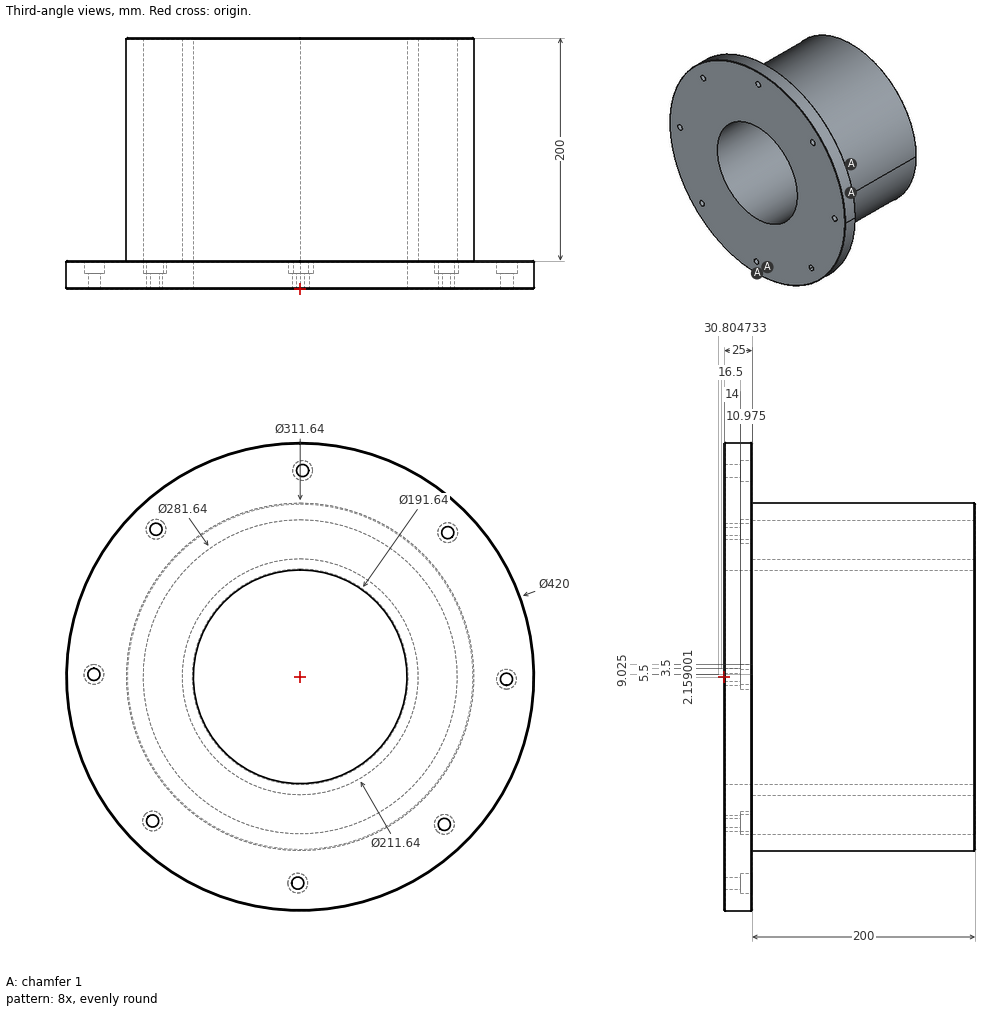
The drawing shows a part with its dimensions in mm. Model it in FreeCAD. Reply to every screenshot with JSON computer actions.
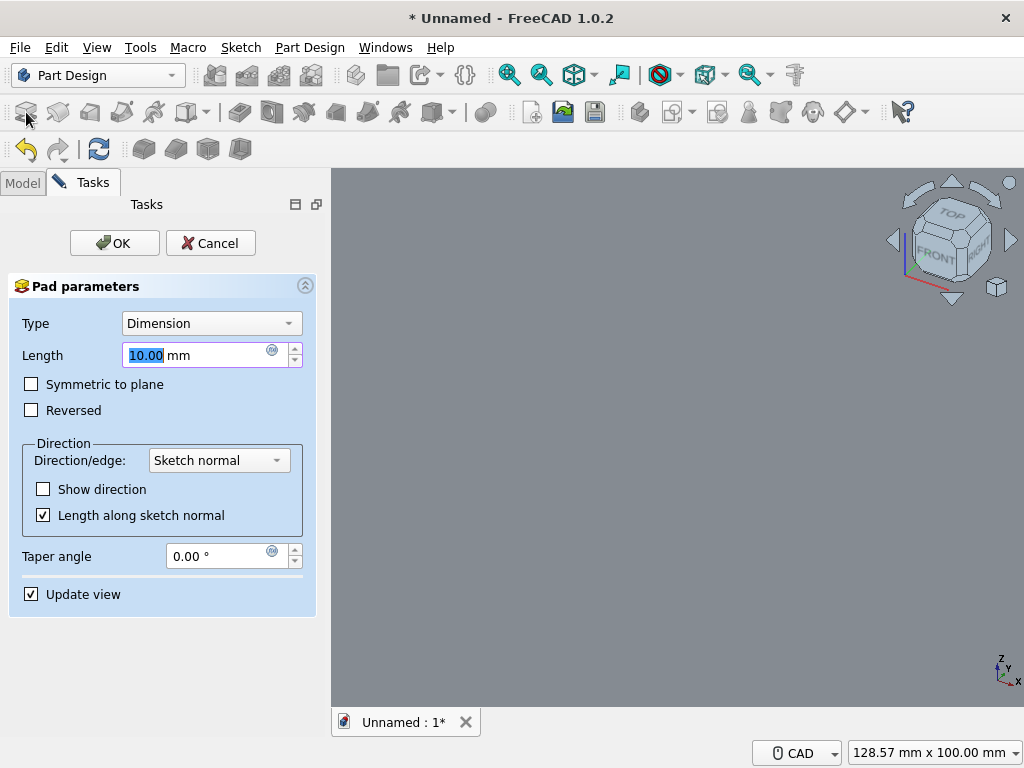
{"action": "type", "text": "25"}
{"action": "key", "text": "Tab"}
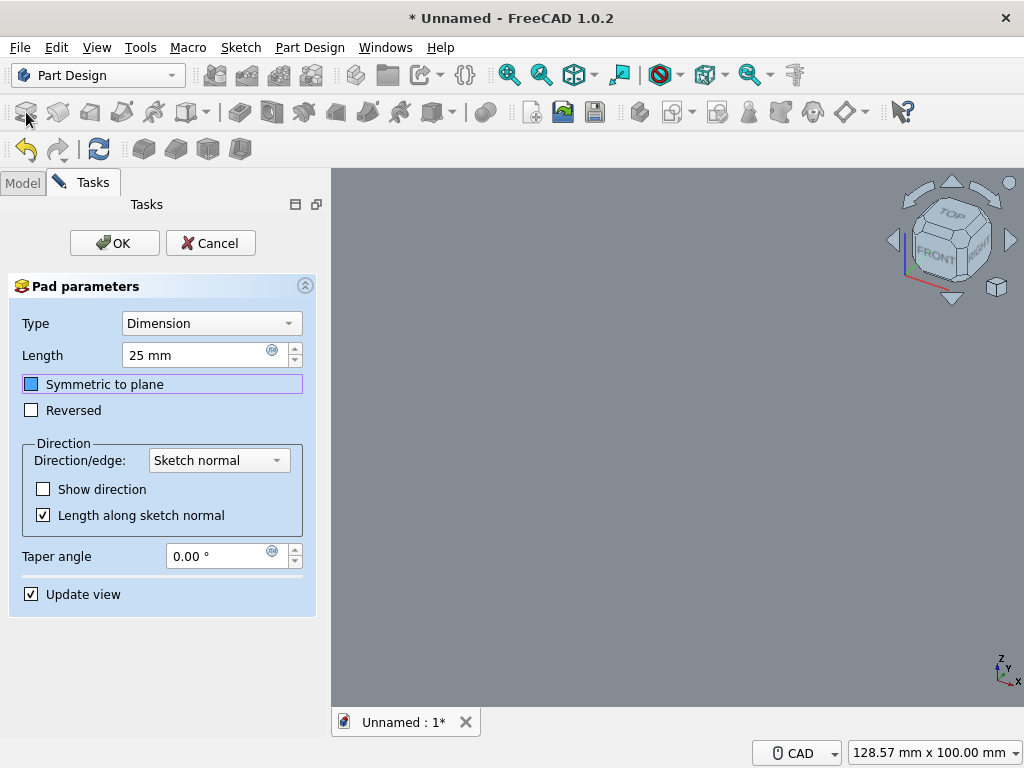
{"action": "left_click", "coordinate": [30, 410]}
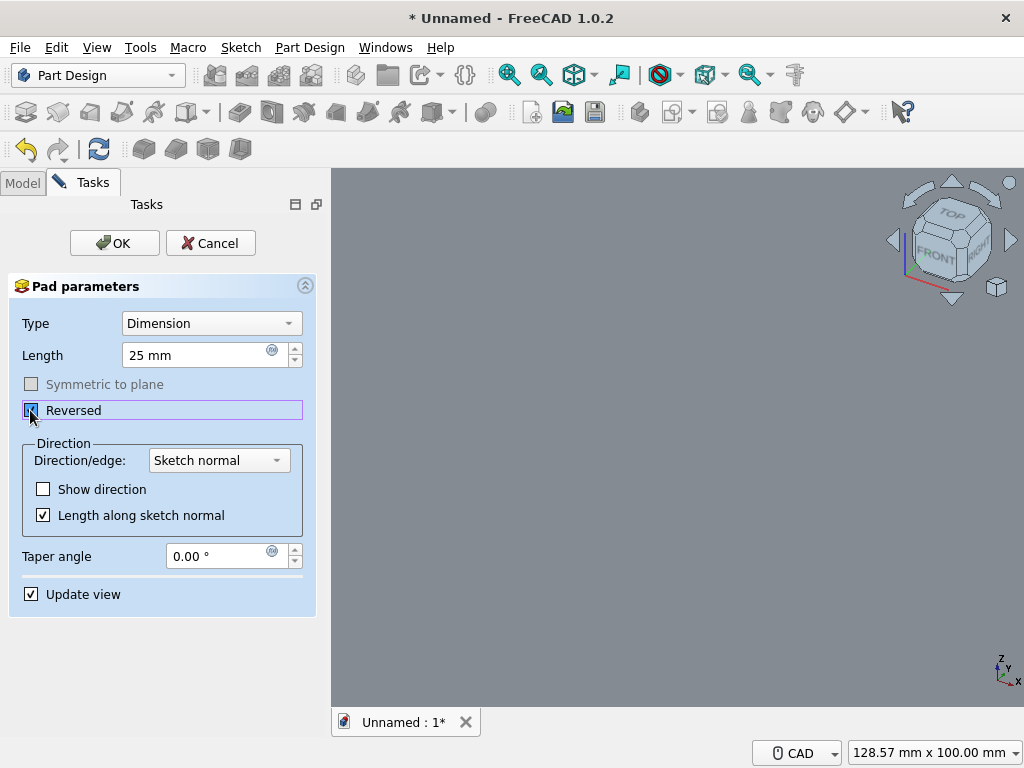
{"action": "left_click", "coordinate": [115, 243]}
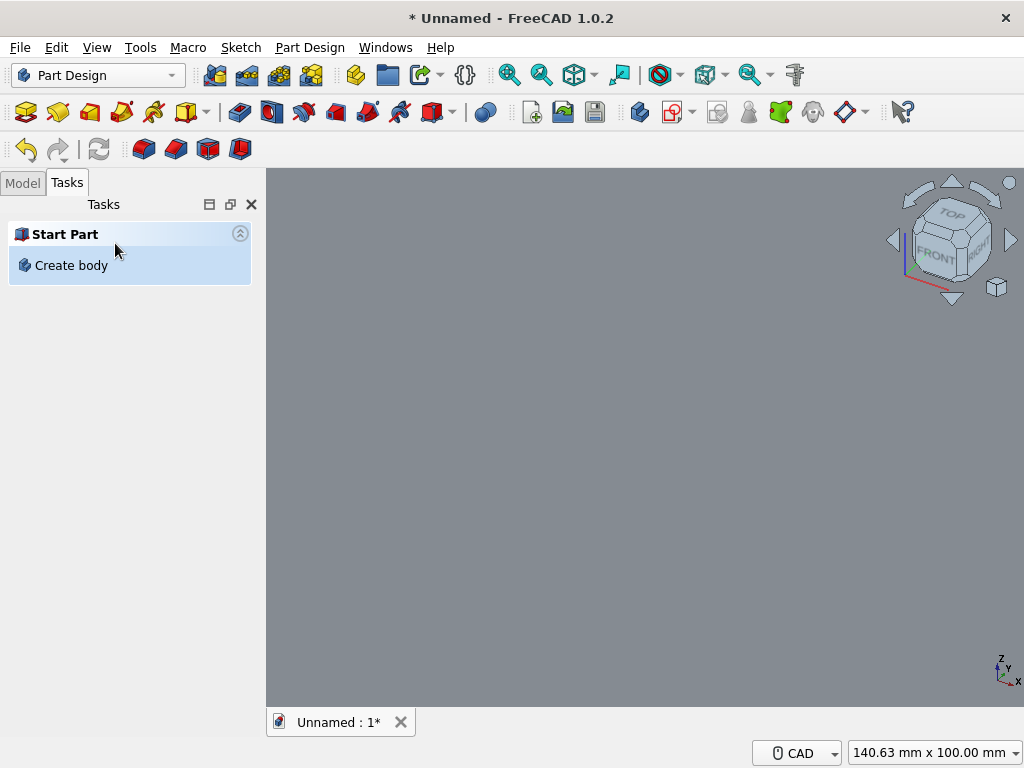
{"action": "key", "text": "v f"}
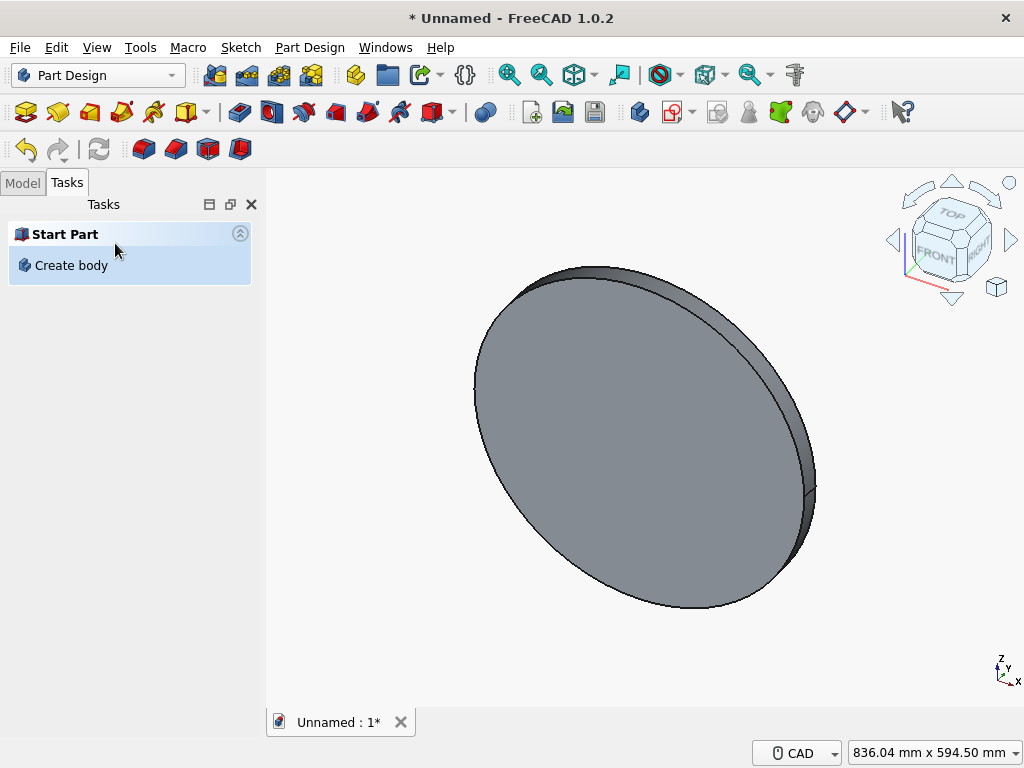
{"action": "key", "text": "4"}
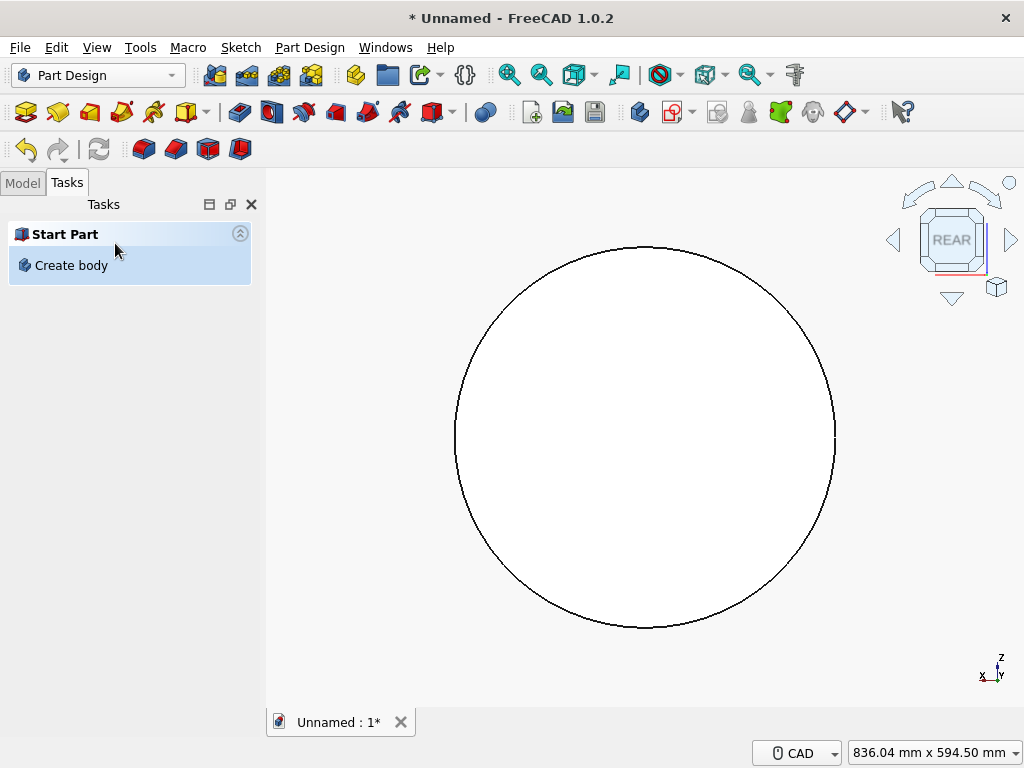
{"action": "left_click", "coordinate": [645, 436]}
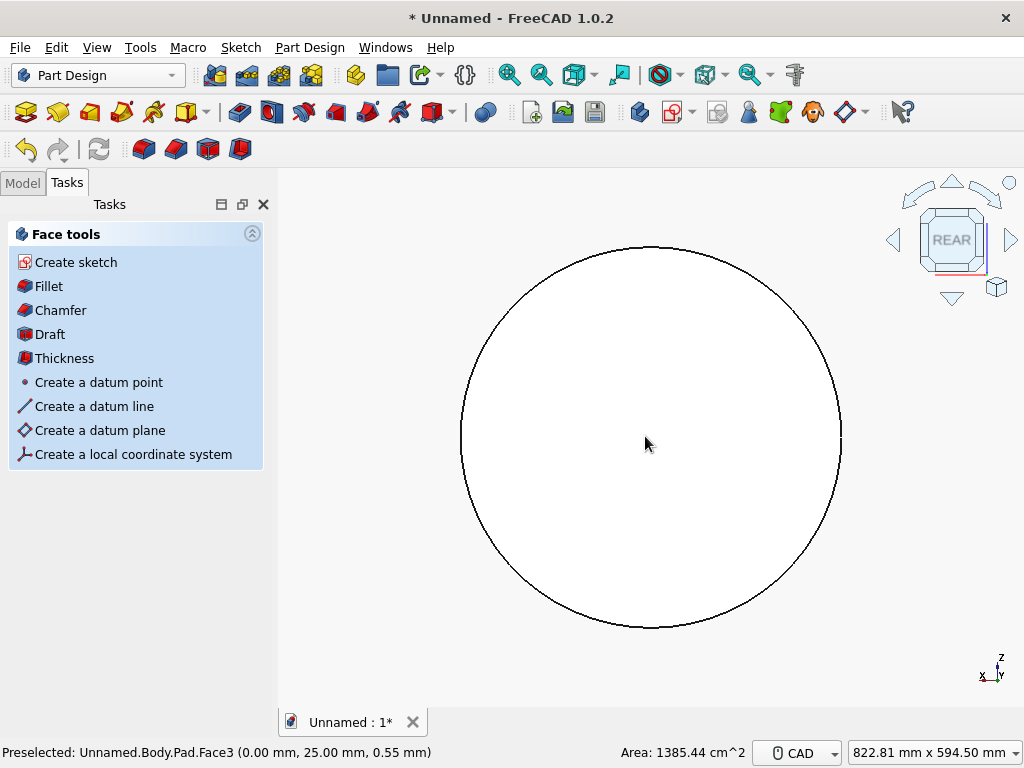
{"action": "left_click", "coordinate": [672, 112]}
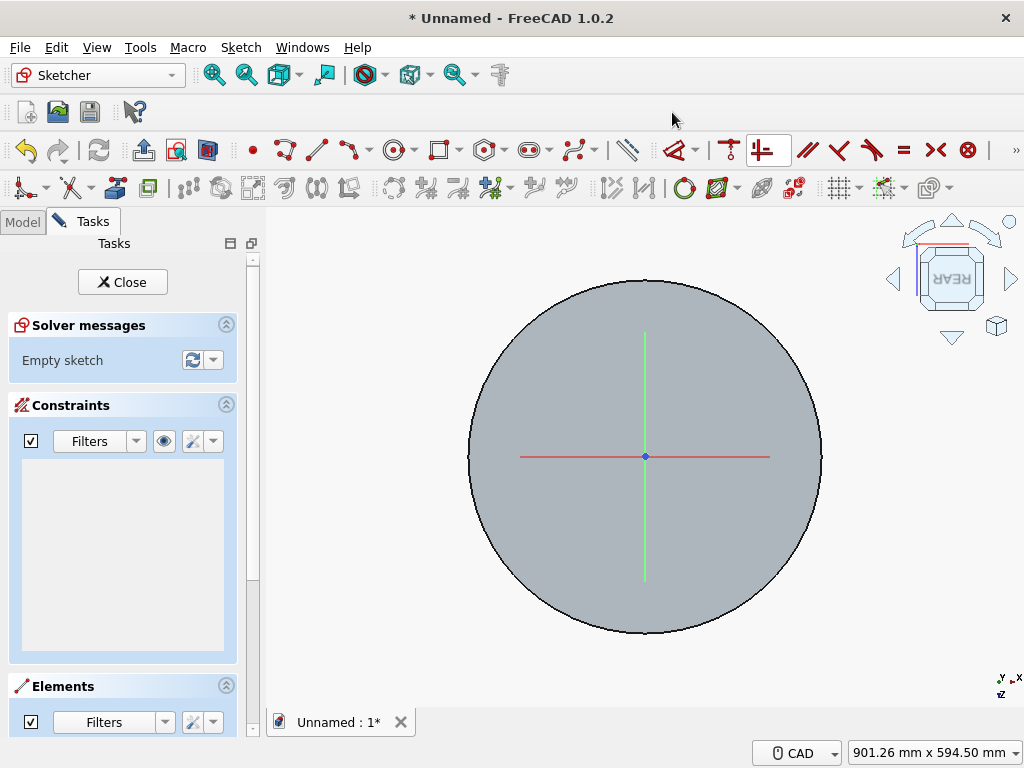
{"action": "scroll", "coordinate": [728, 457], "scroll_direction": "up", "scroll_amount": 3}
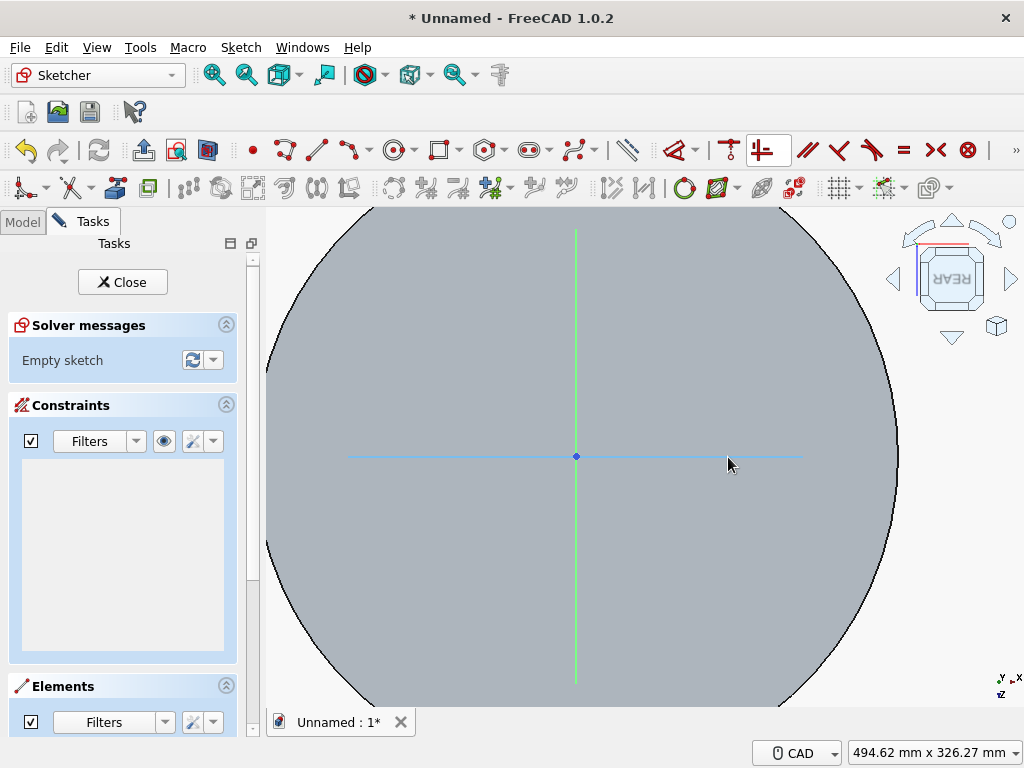
{"action": "left_click", "coordinate": [394, 150]}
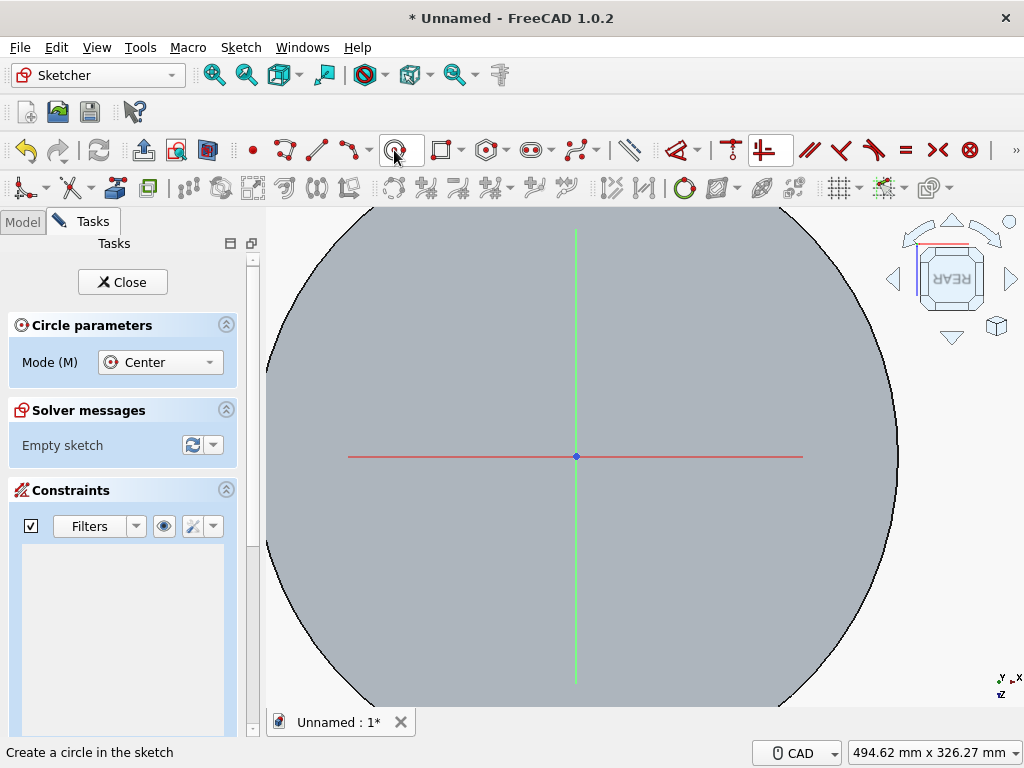
{"action": "left_click", "coordinate": [576, 457]}
{"action": "left_click", "coordinate": [680, 353]}
{"action": "key", "text": "Escape"}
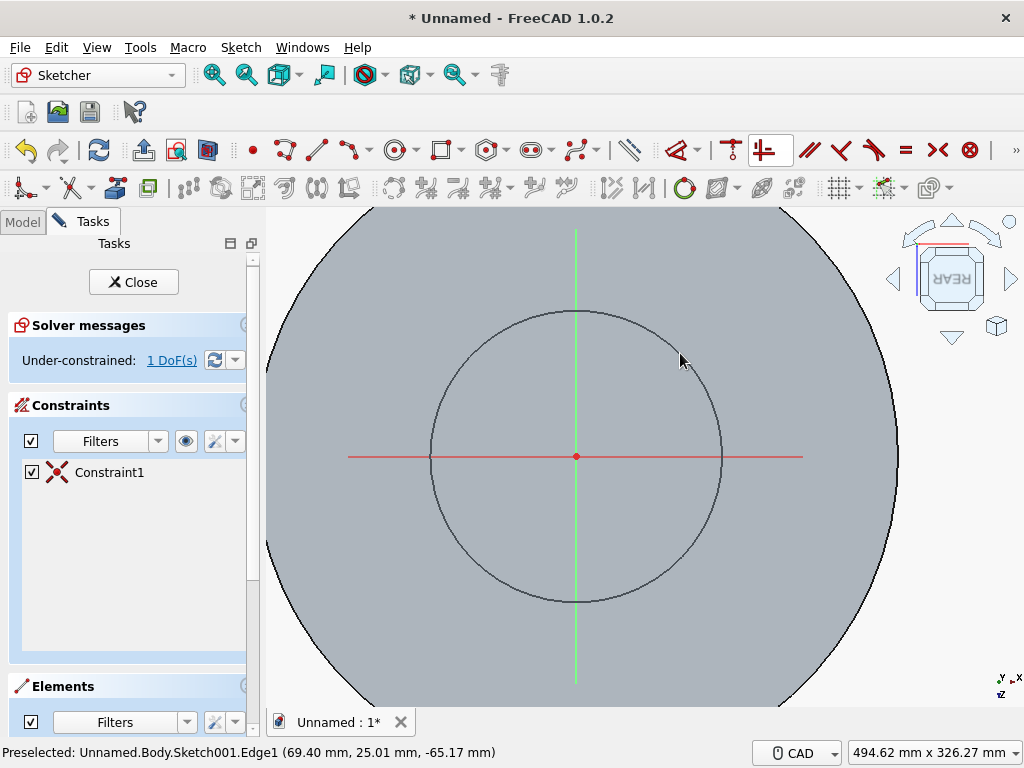
{"action": "left_click", "coordinate": [676, 150]}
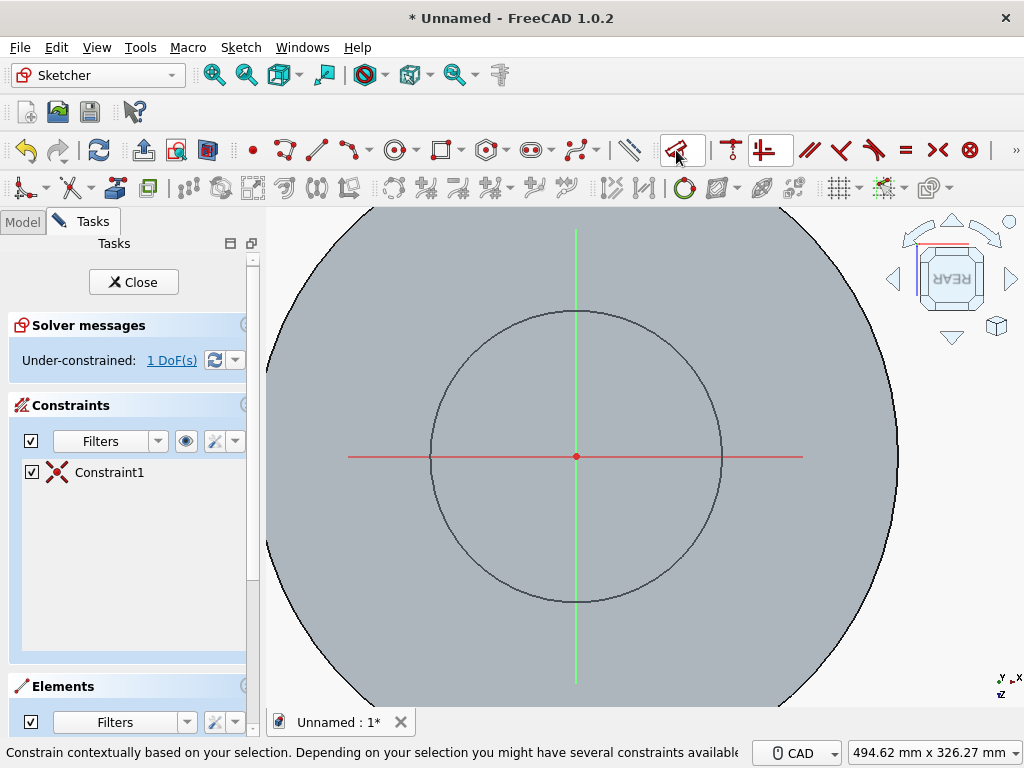
{"action": "left_click", "coordinate": [679, 353]}
{"action": "left_click", "coordinate": [702, 330]}